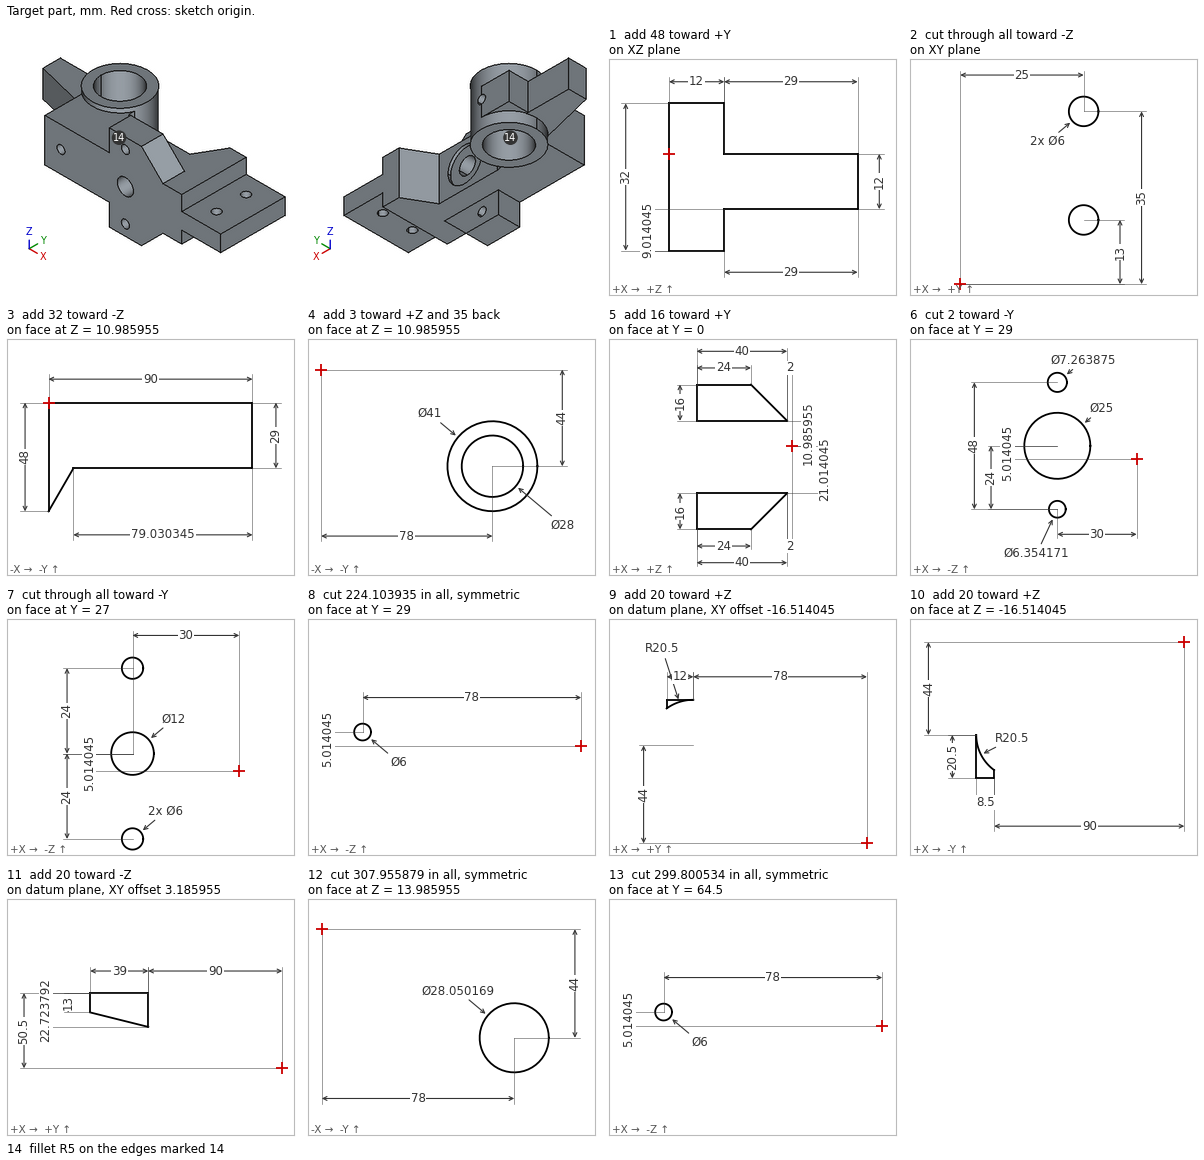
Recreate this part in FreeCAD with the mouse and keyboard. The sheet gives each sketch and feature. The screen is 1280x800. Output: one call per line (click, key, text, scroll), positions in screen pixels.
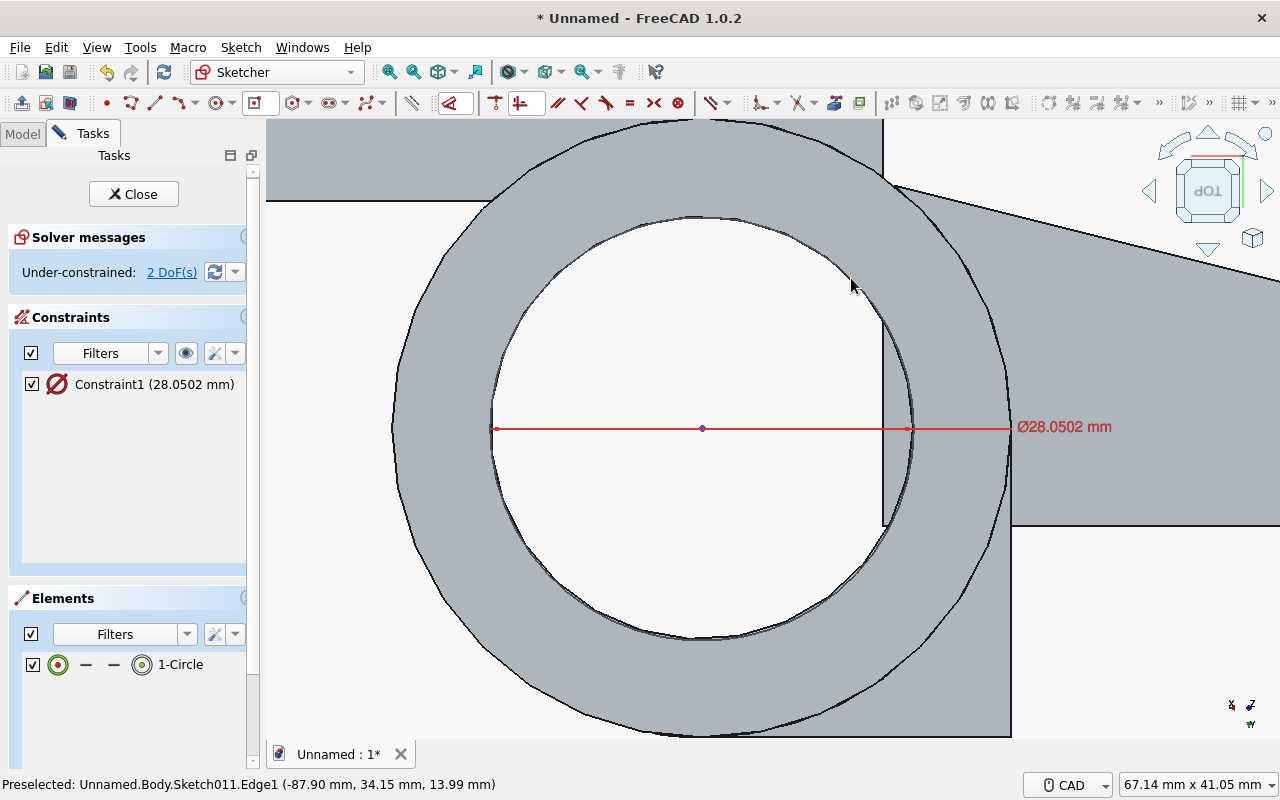
click(702, 429)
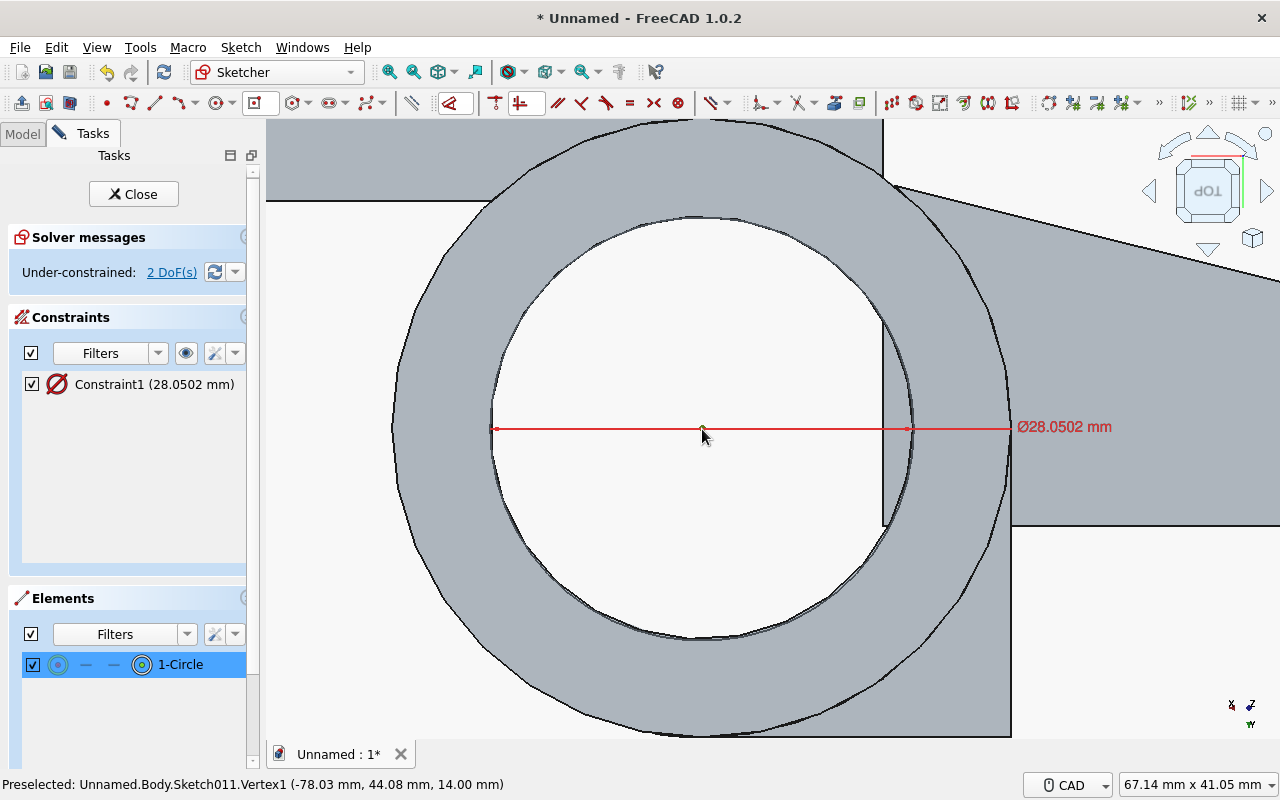
key(l)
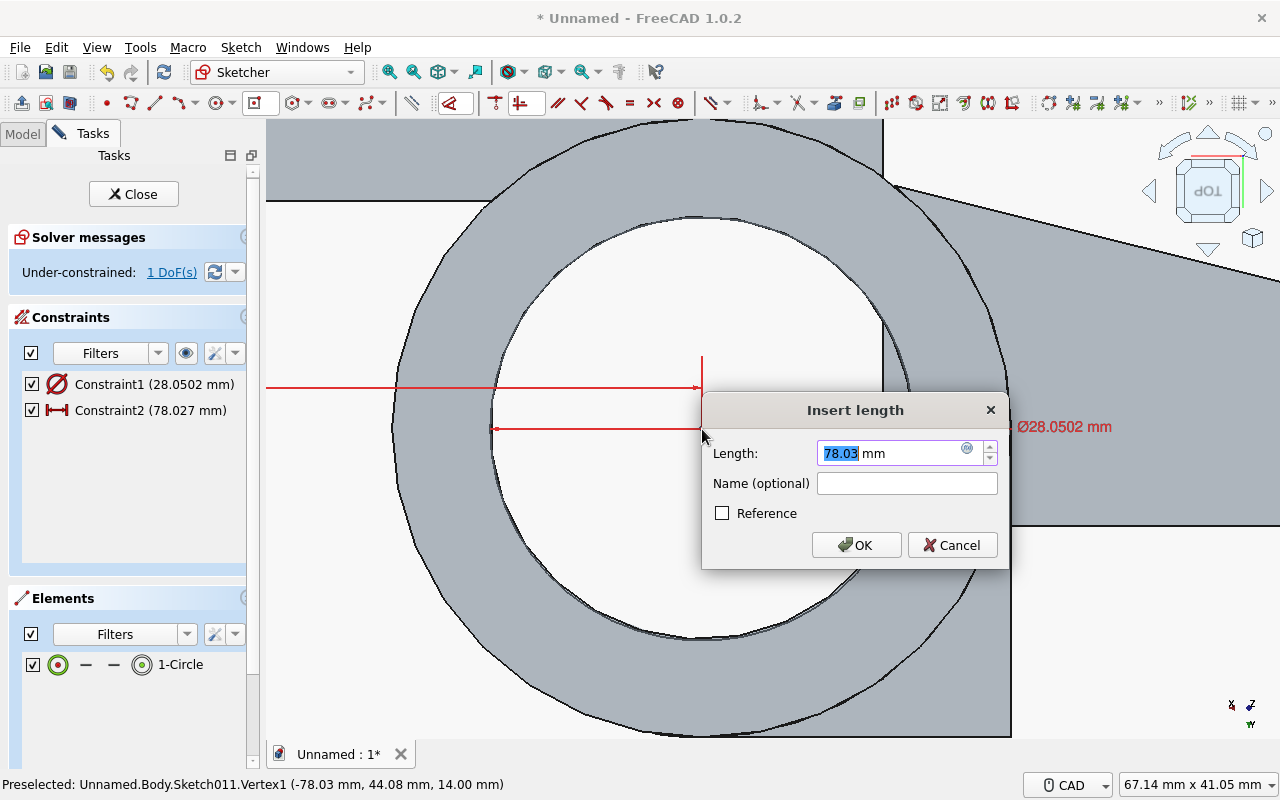
text(78)
key(Return)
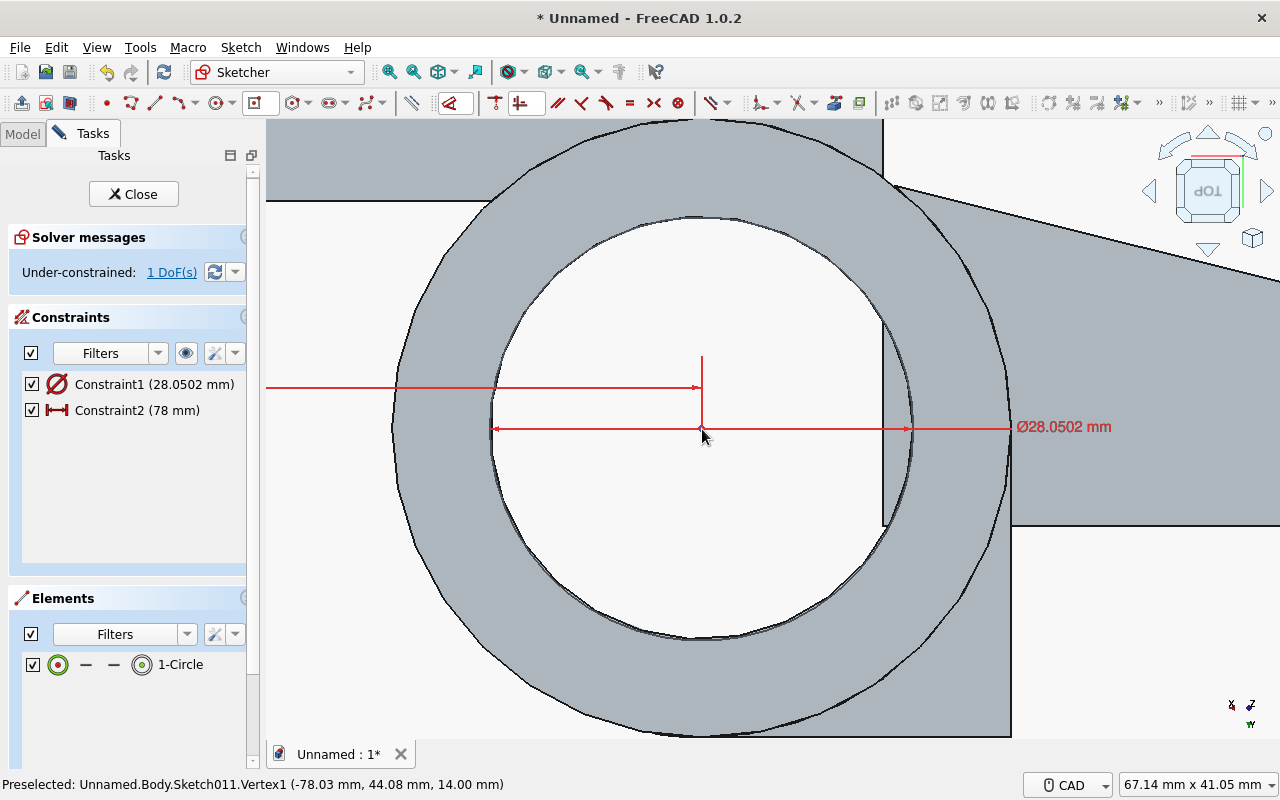
click(702, 429)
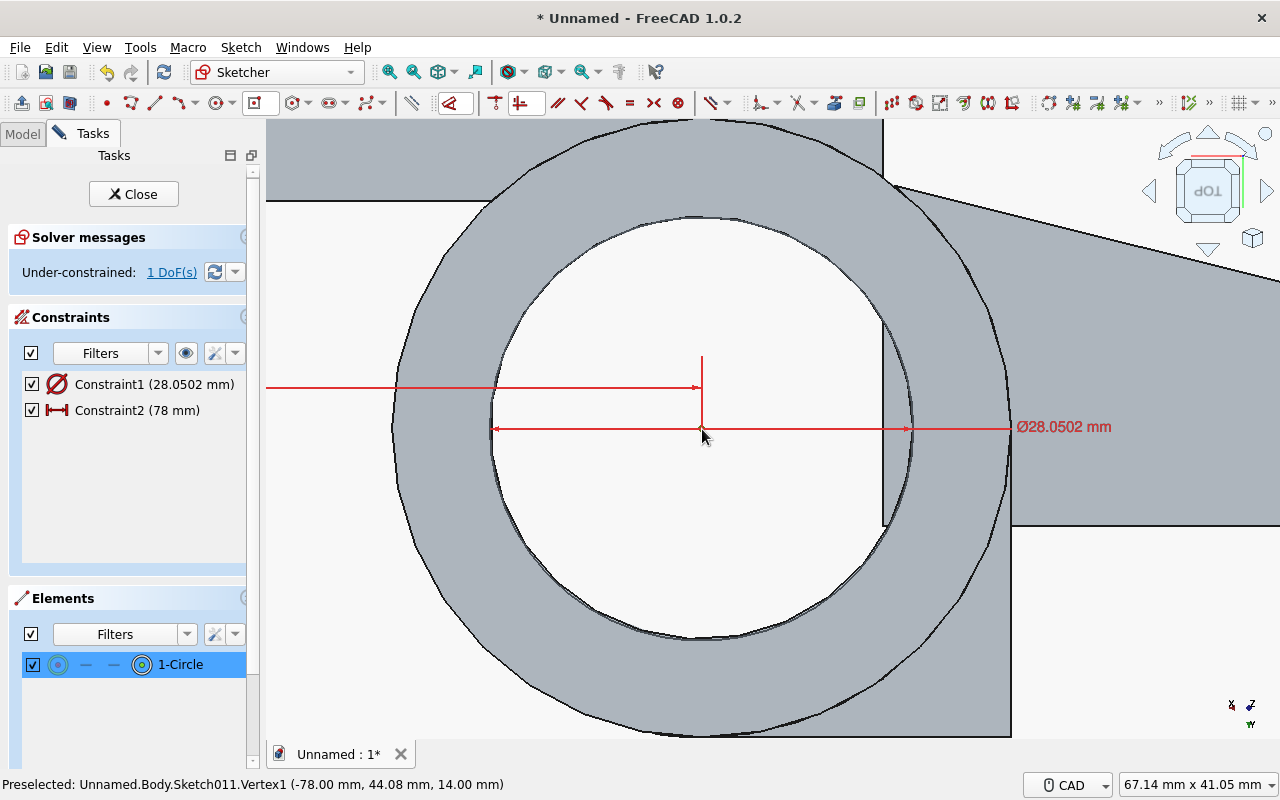
click(468, 104)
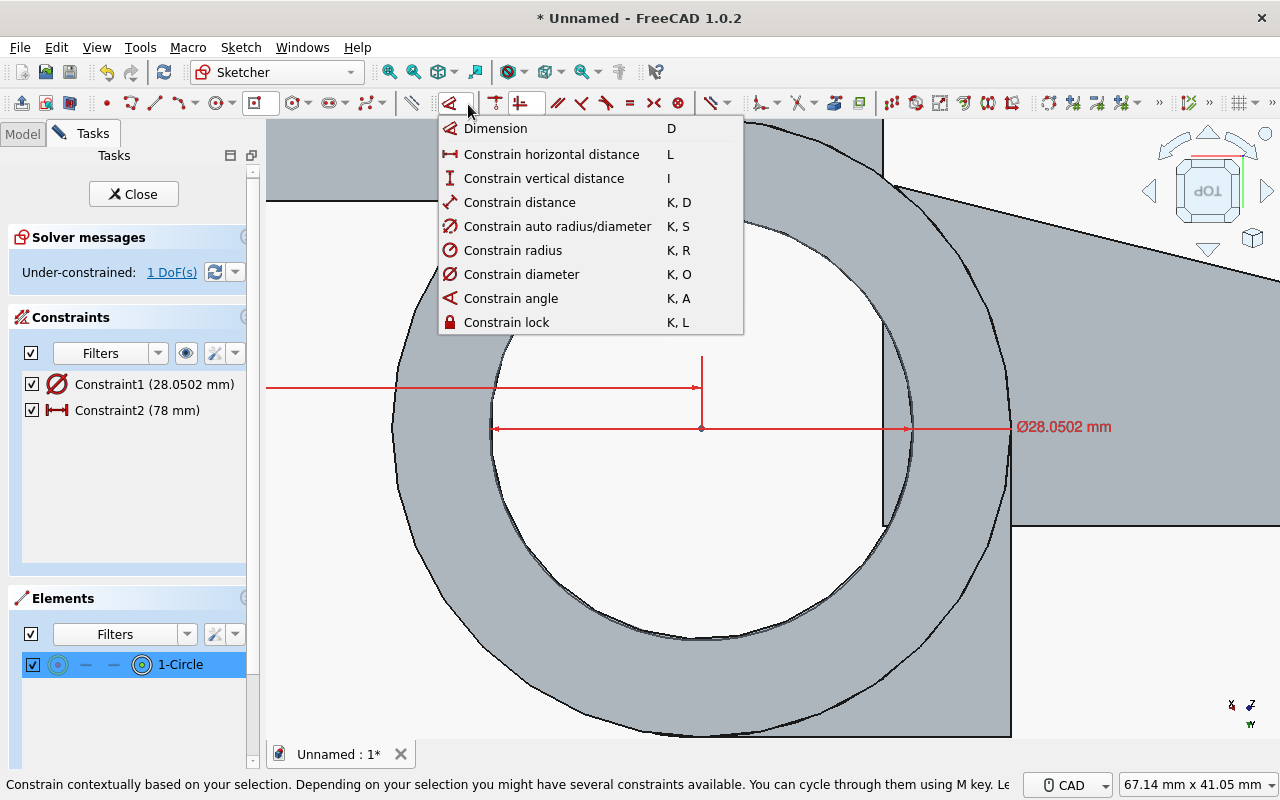
click(591, 178)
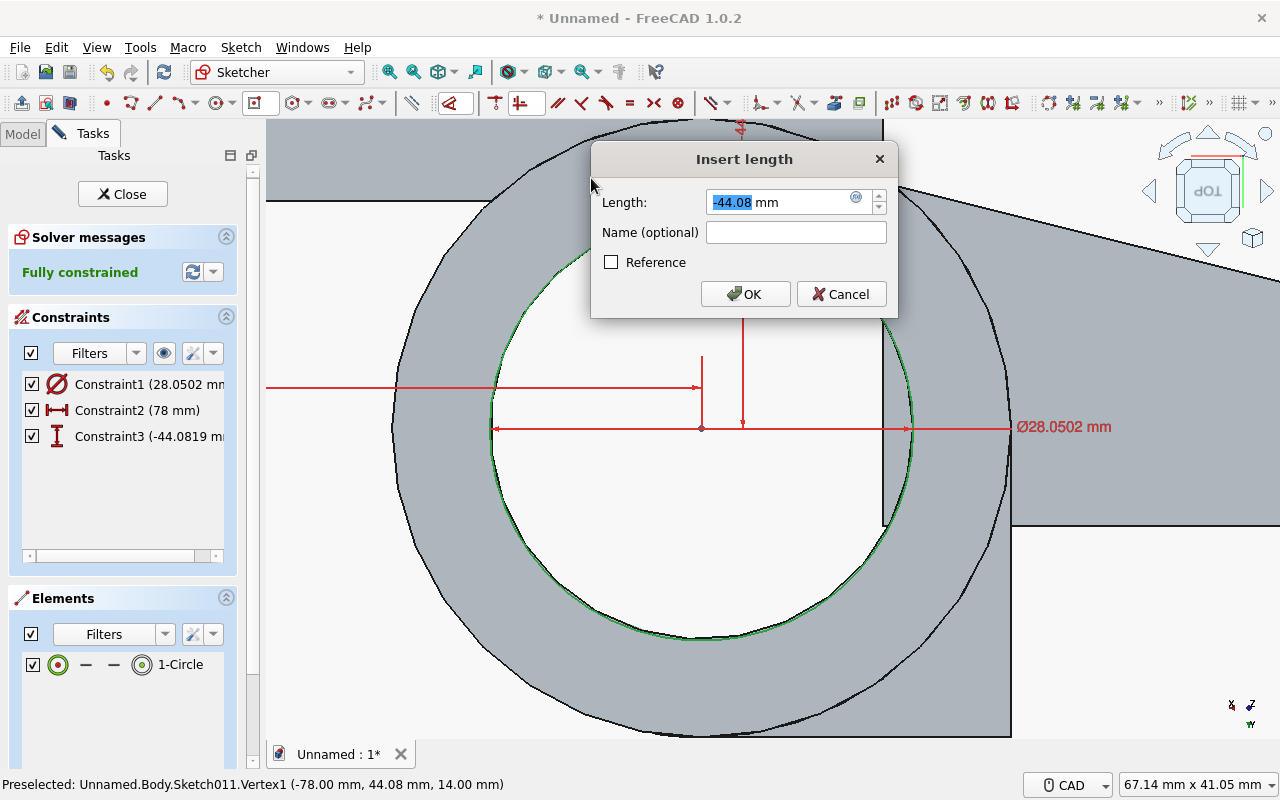
text(-44)
key(Return)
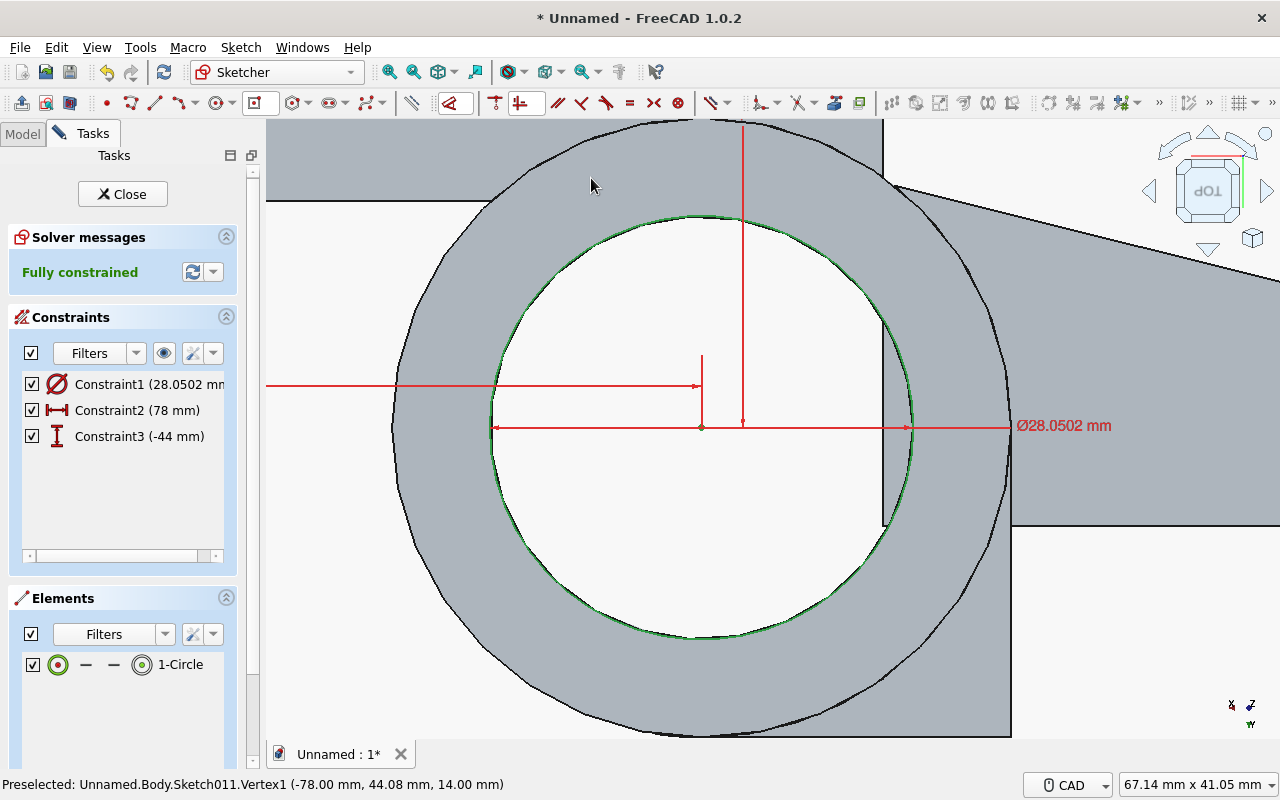
click(123, 194)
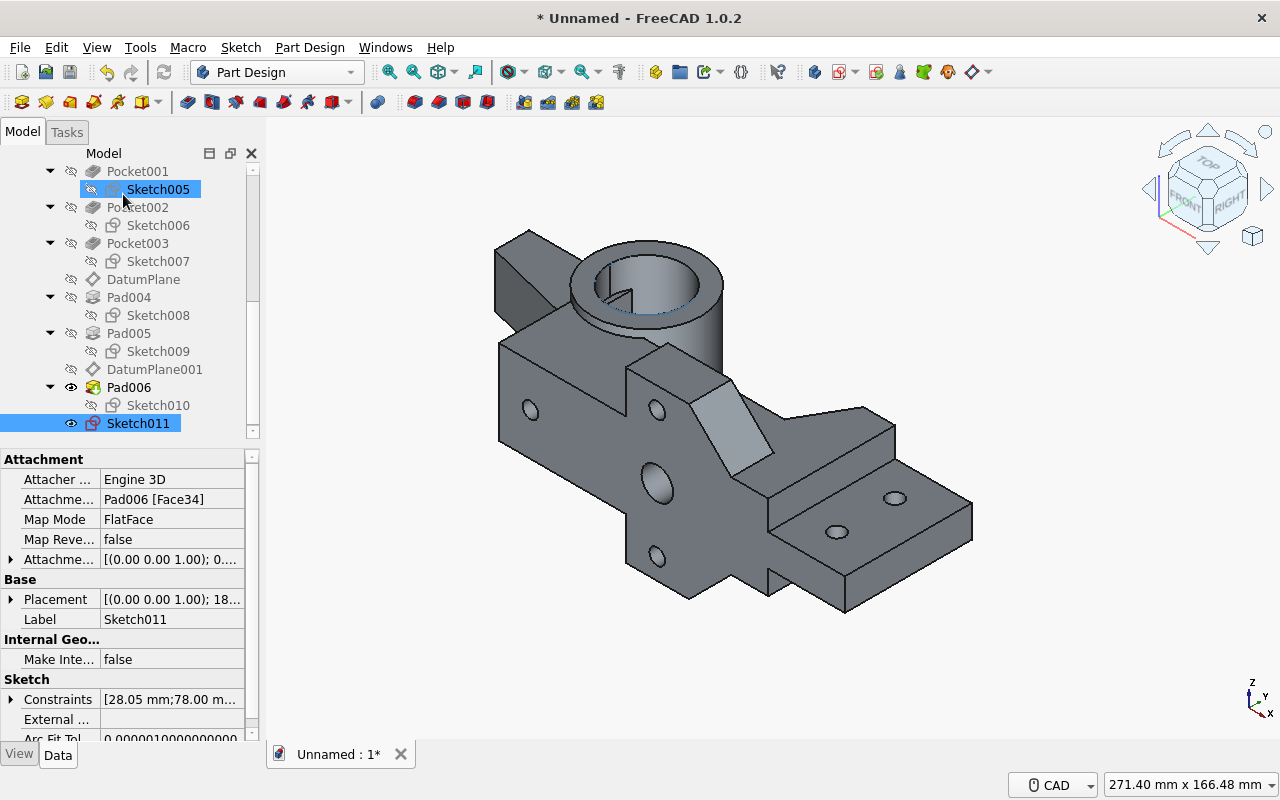
click(188, 102)